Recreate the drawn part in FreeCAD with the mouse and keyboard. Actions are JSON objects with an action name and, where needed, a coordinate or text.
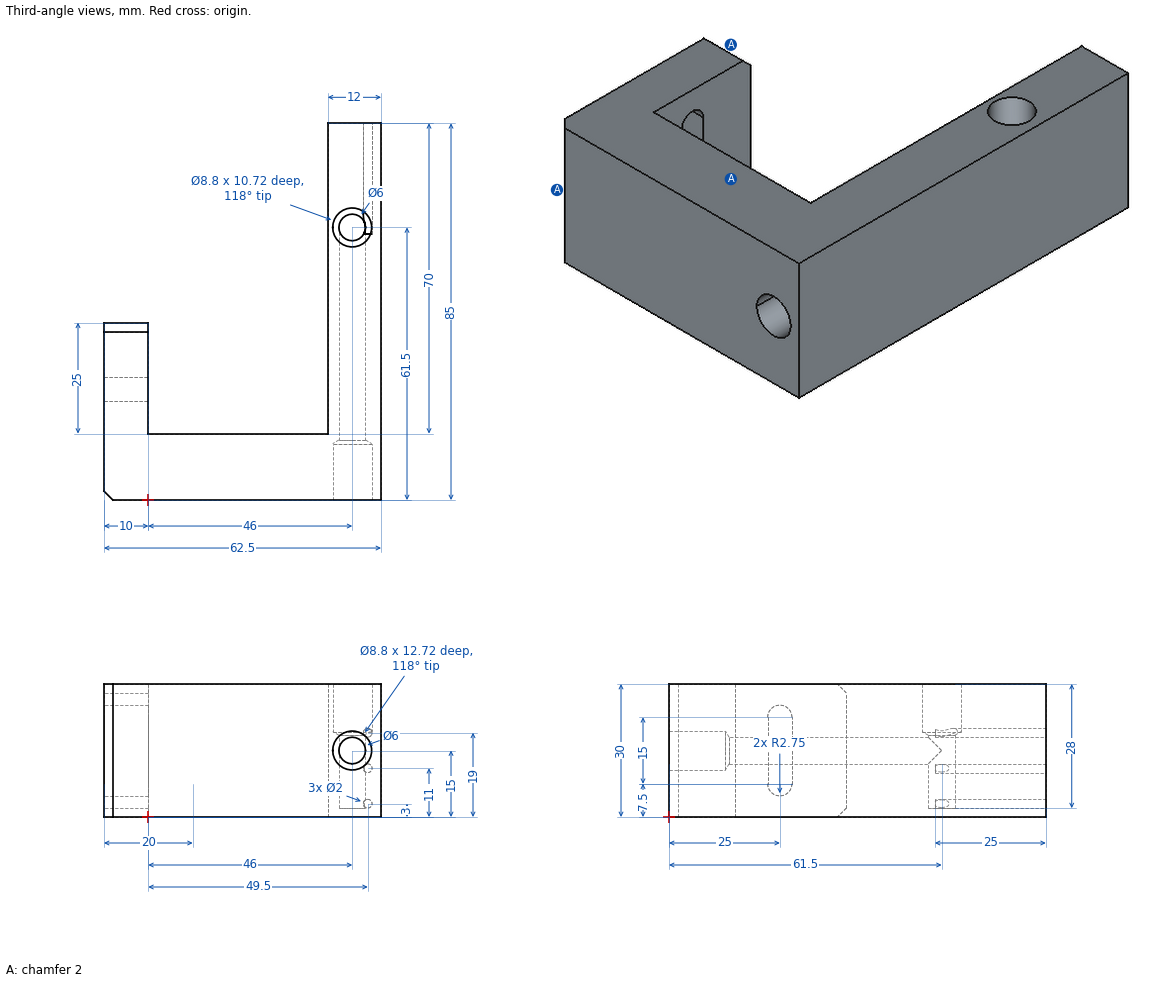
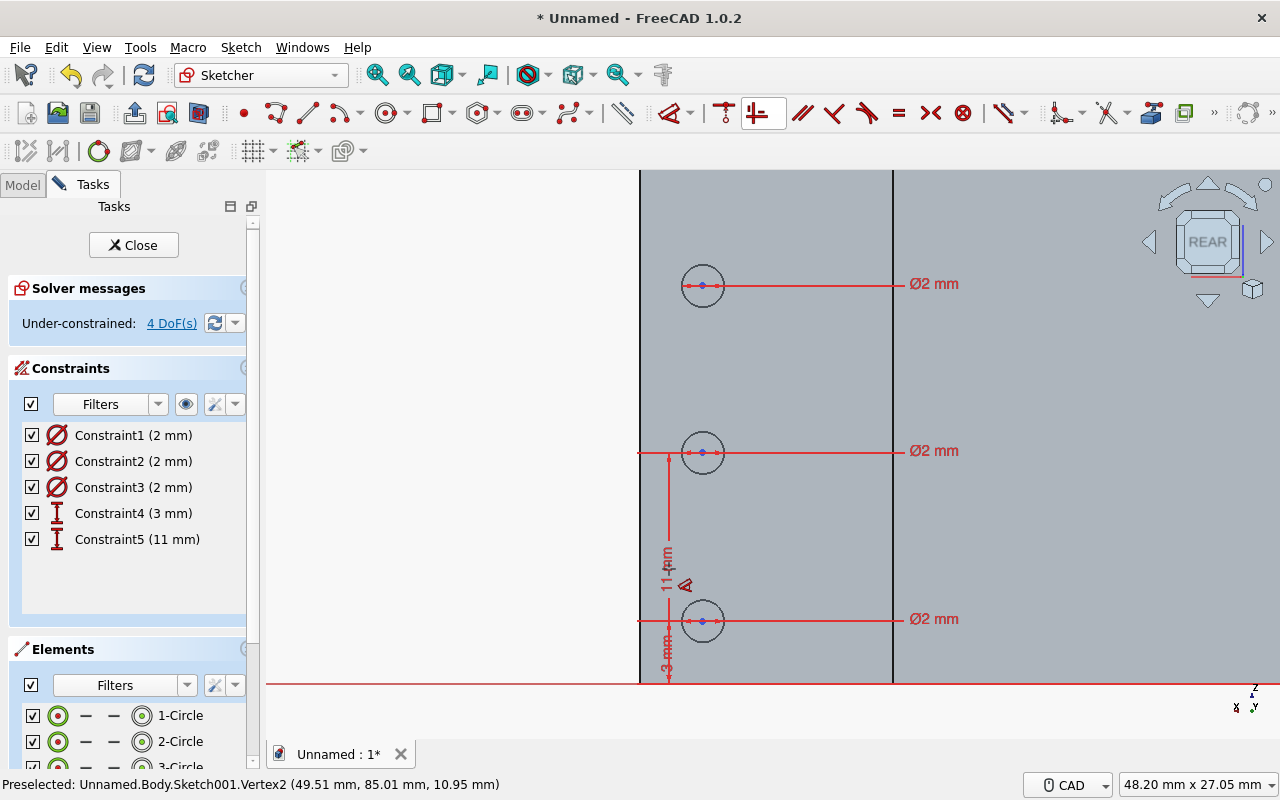
{"action": "left_click", "coordinate": [703, 286]}
{"action": "left_click", "coordinate": [669, 485]}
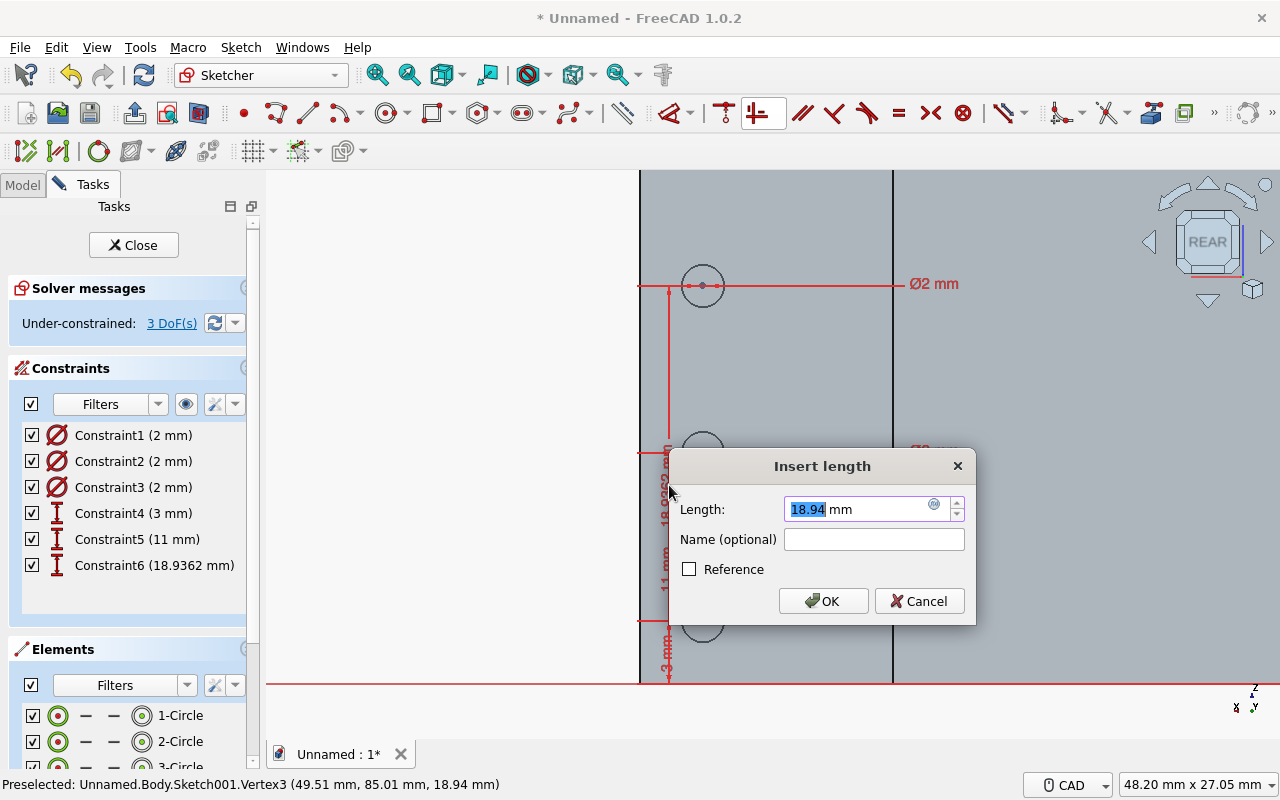
{"action": "type", "text": "19"}
{"action": "key", "text": "Return"}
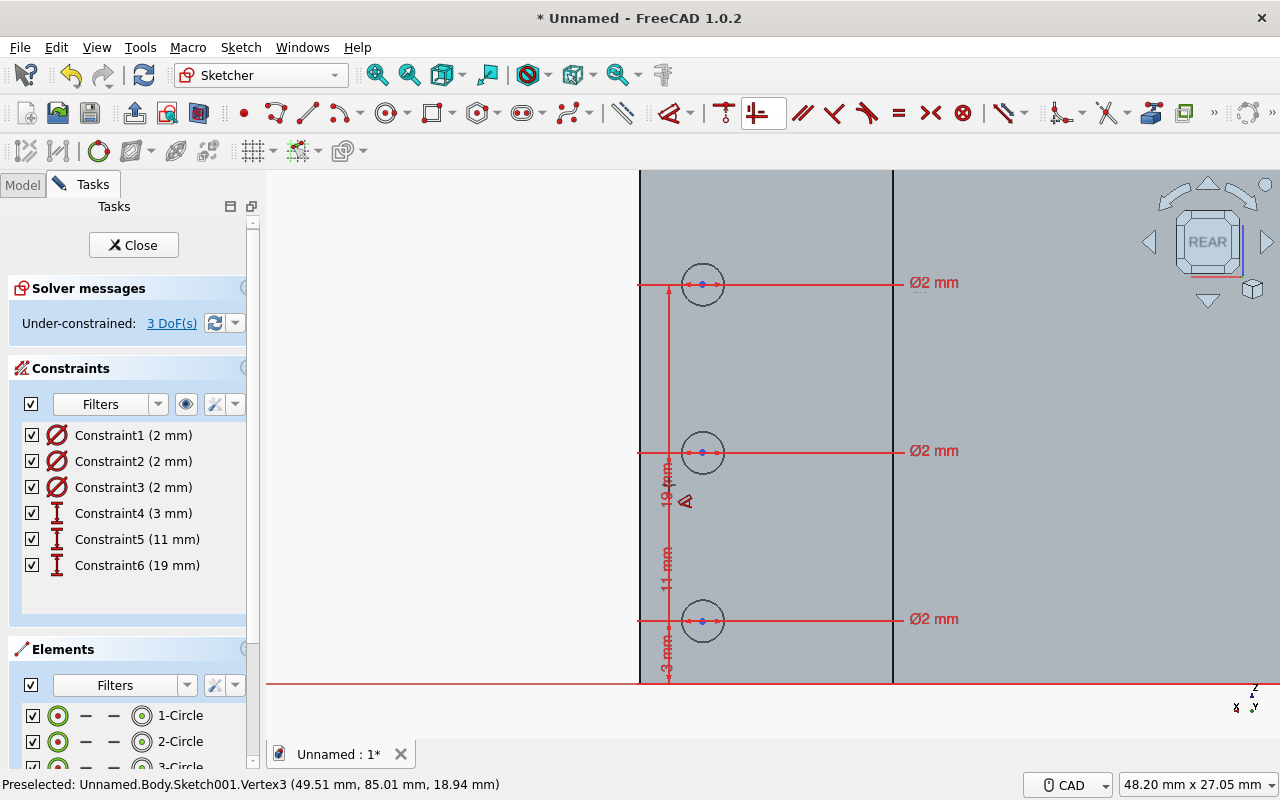
{"action": "left_click", "coordinate": [703, 621]}
{"action": "left_click", "coordinate": [909, 587]}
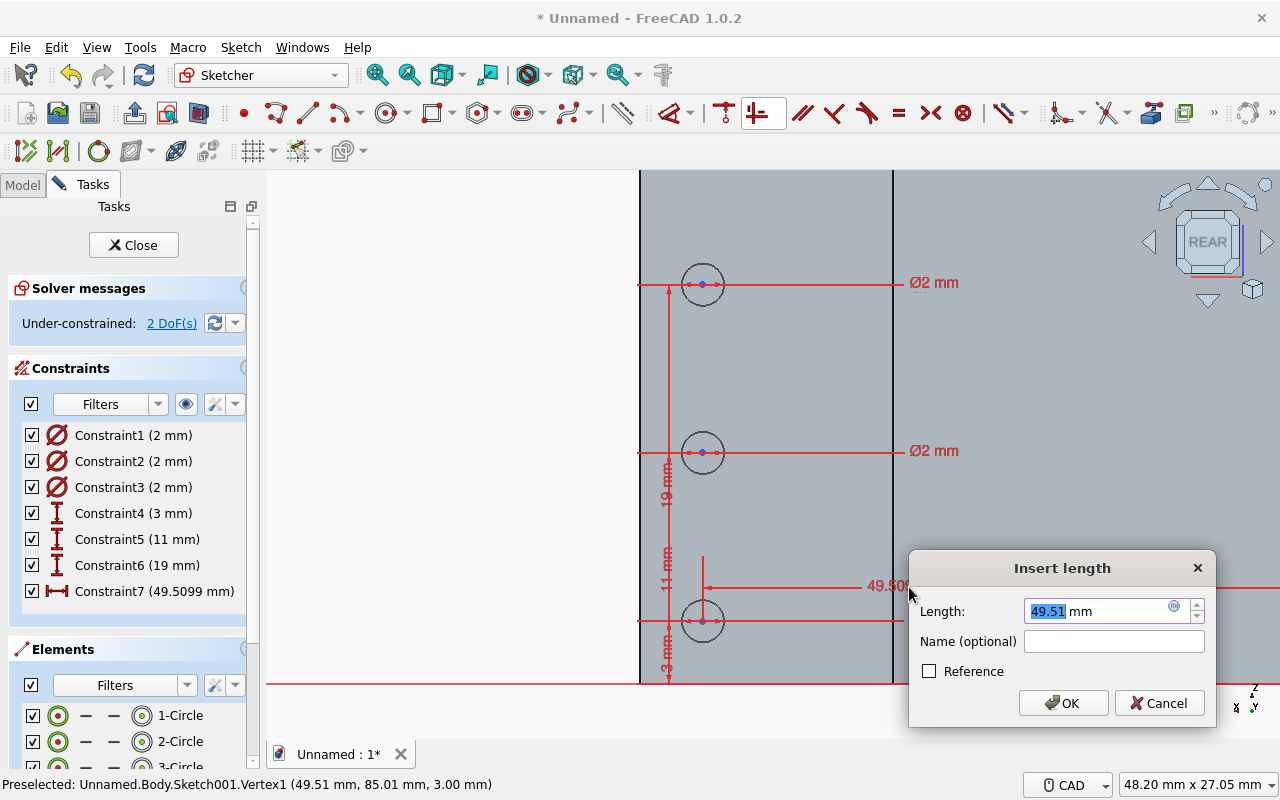
{"action": "type", "text": "49.5"}
{"action": "key", "text": "Return"}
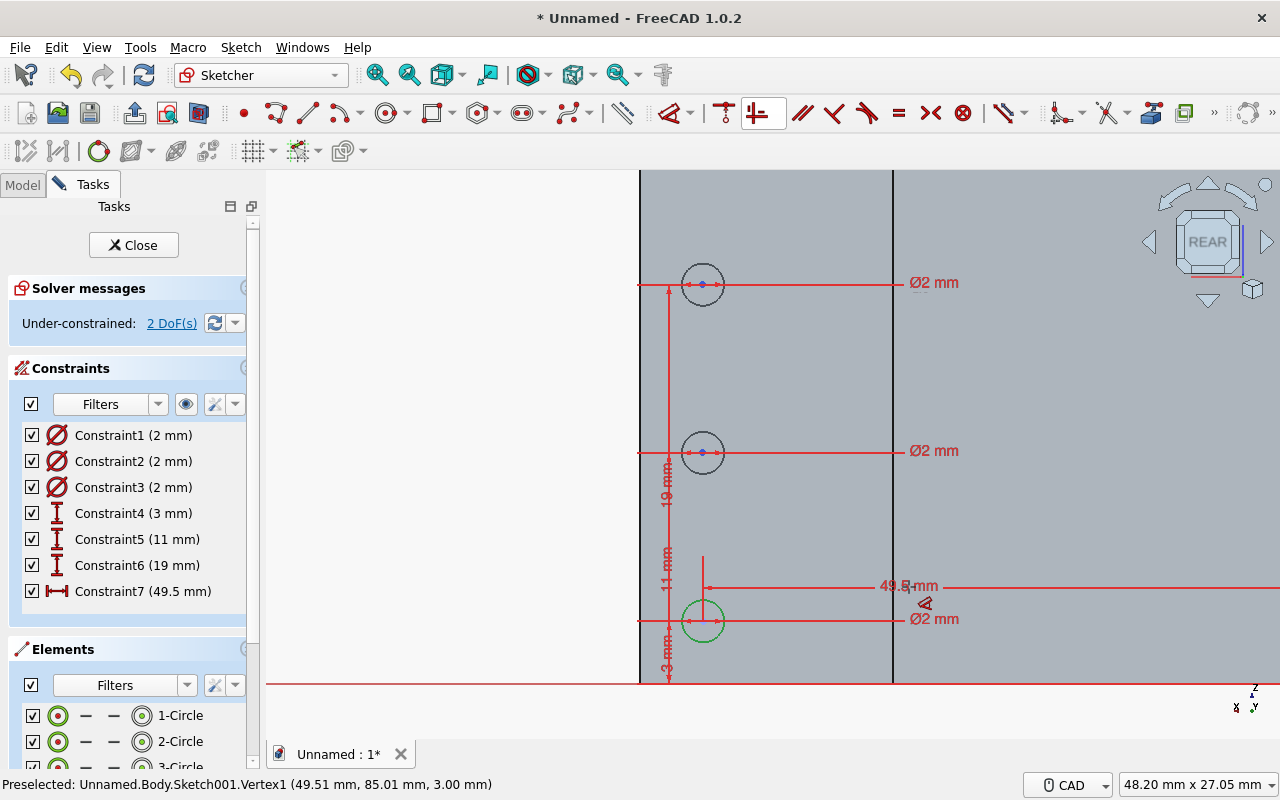
{"action": "left_click", "coordinate": [703, 453]}
{"action": "left_click", "coordinate": [909, 419]}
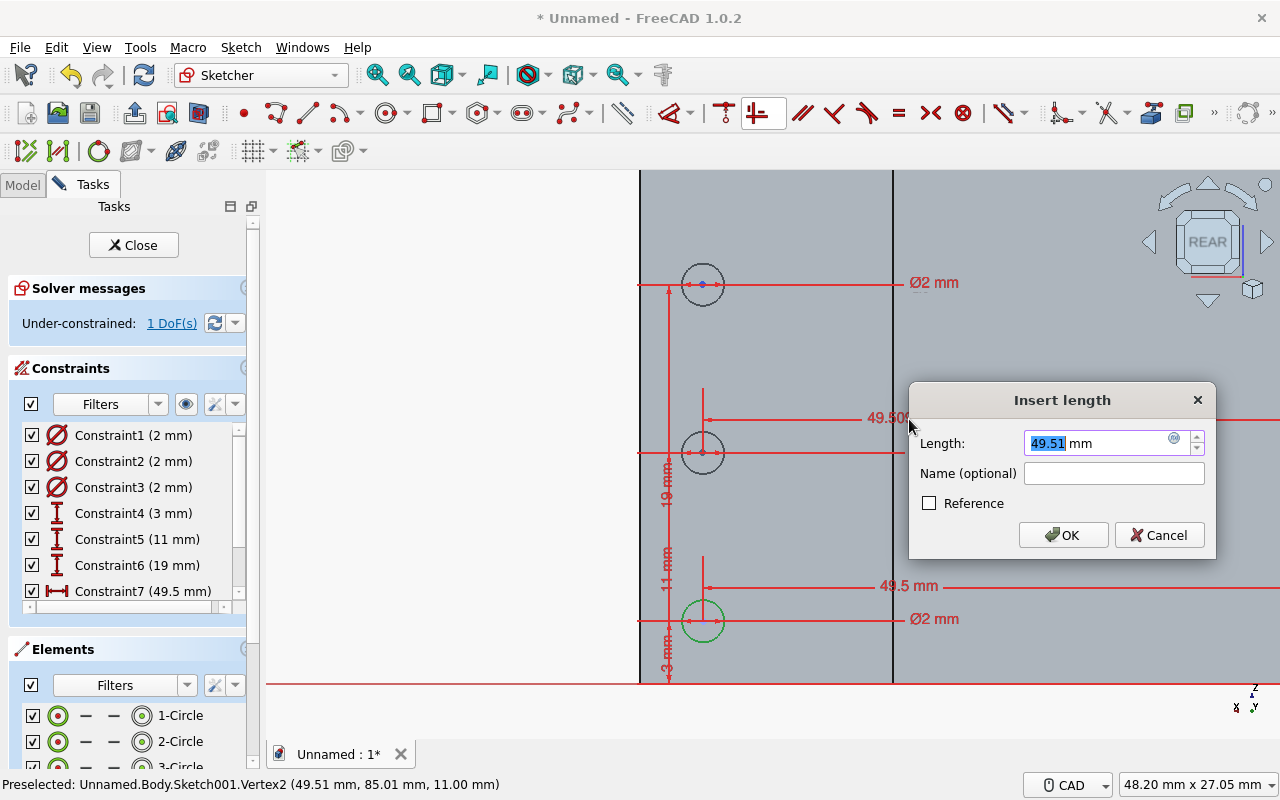
{"action": "type", "text": "49.5"}
{"action": "key", "text": "Return"}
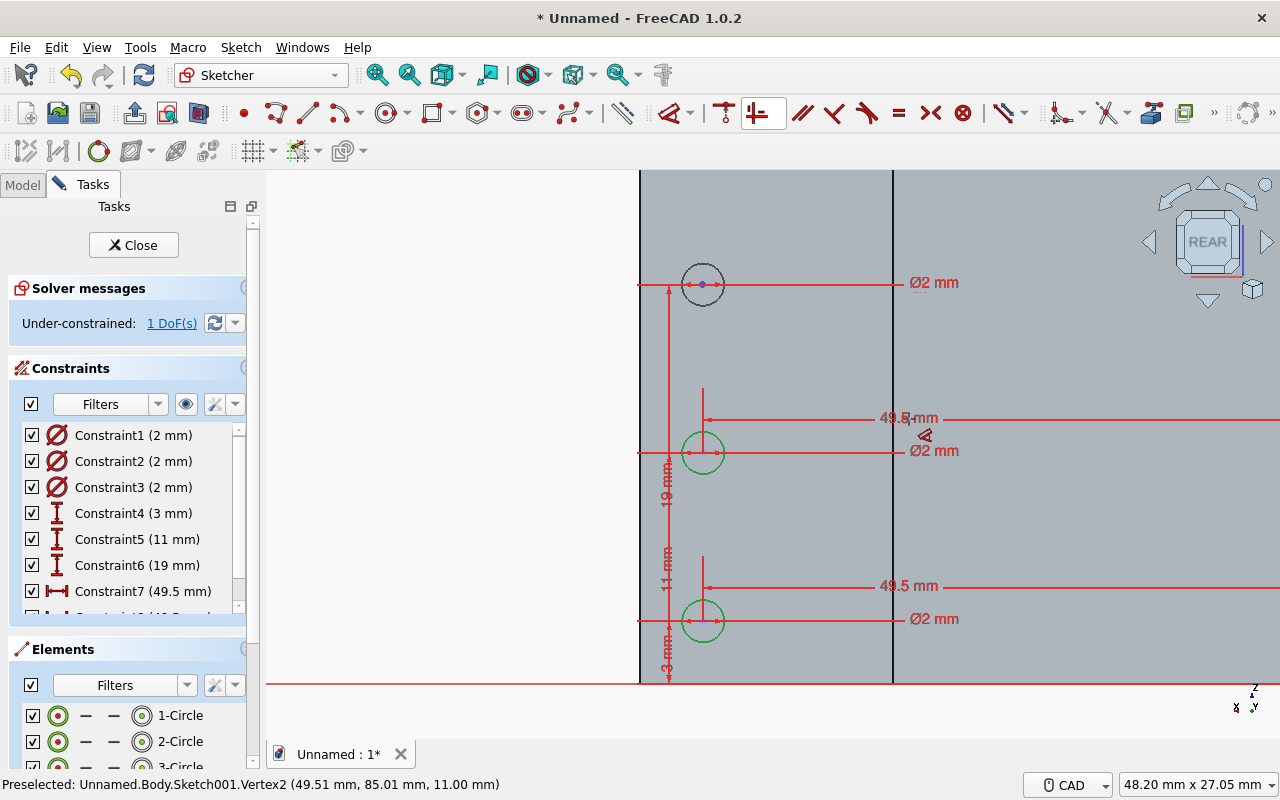
{"action": "left_click", "coordinate": [703, 285]}
{"action": "left_click", "coordinate": [909, 251]}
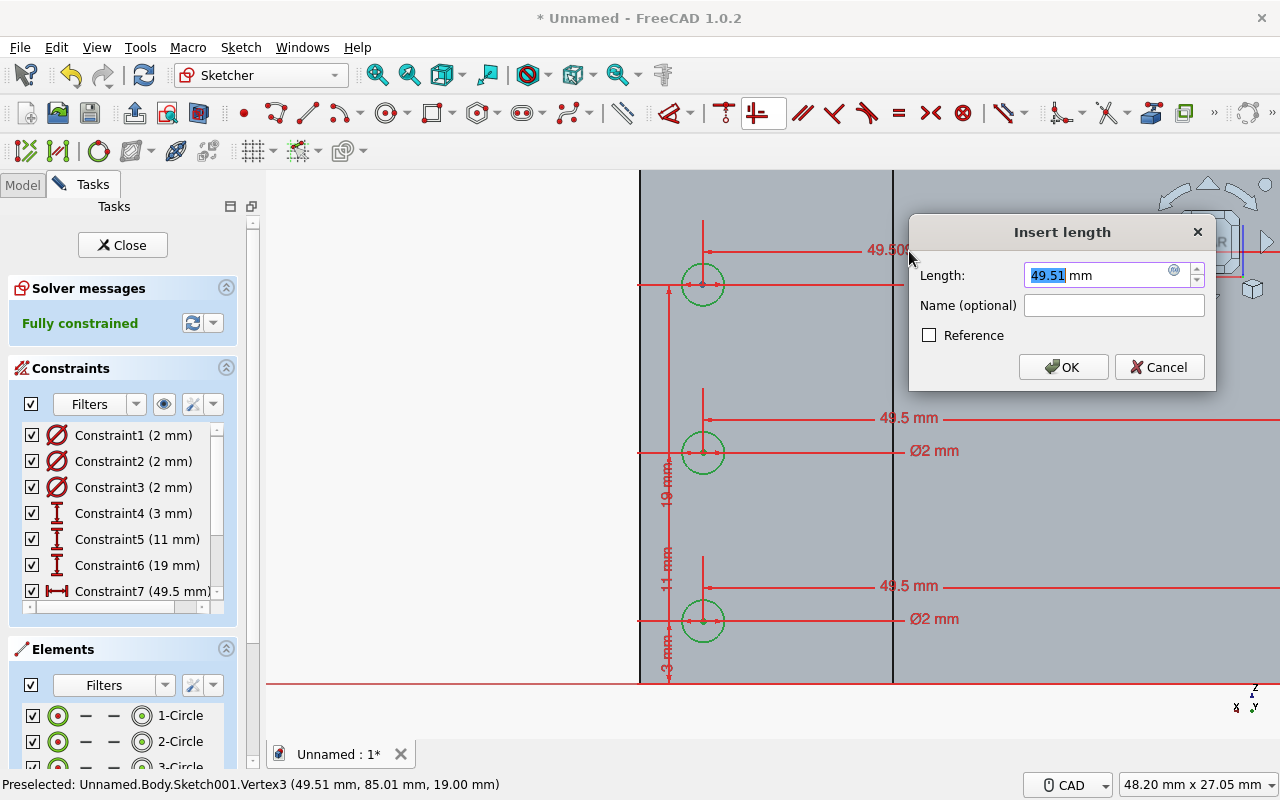
{"action": "type", "text": "49.5"}
{"action": "key", "text": "Return"}
{"action": "key", "text": "Escape"}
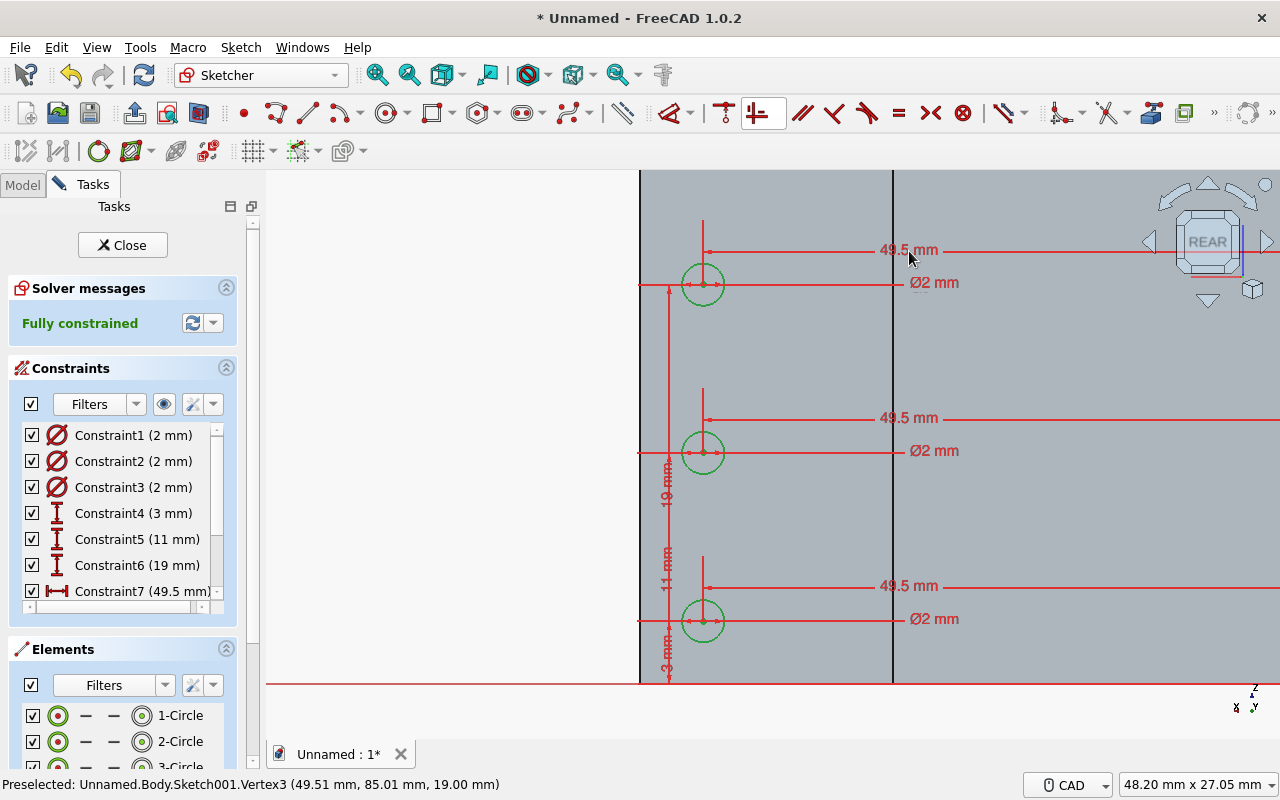
{"action": "left_click", "coordinate": [123, 245]}